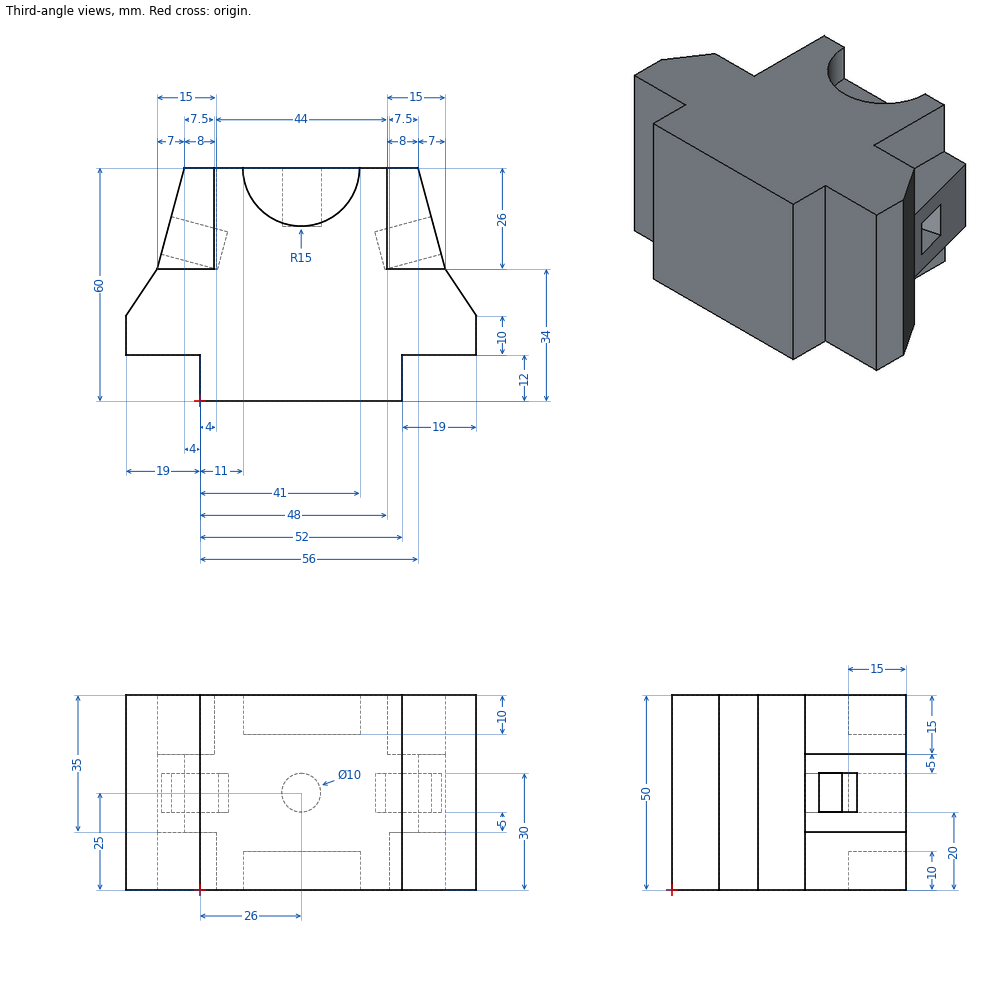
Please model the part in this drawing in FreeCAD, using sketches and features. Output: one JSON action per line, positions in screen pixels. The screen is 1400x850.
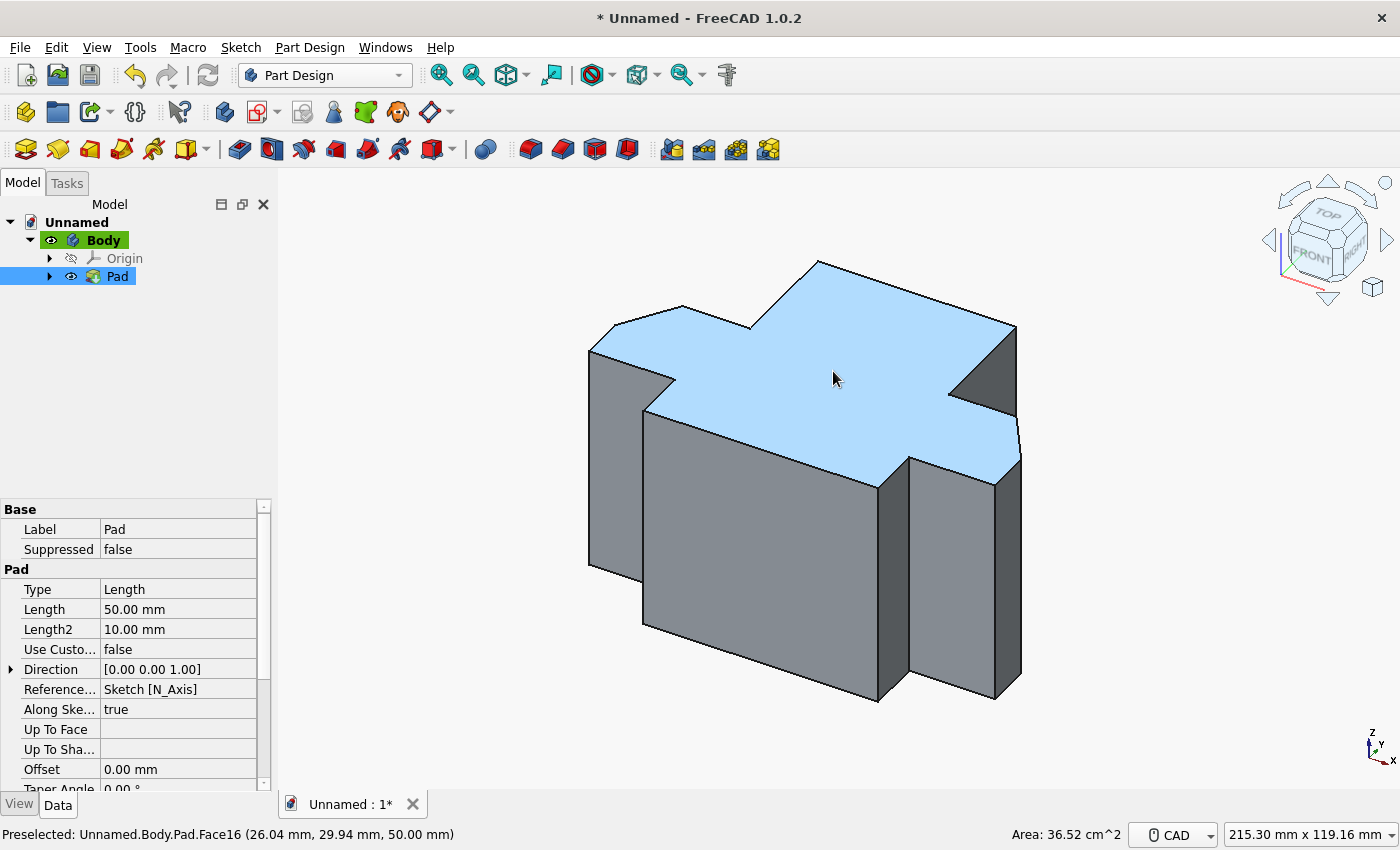
{"action": "left_click", "coordinate": [258, 112]}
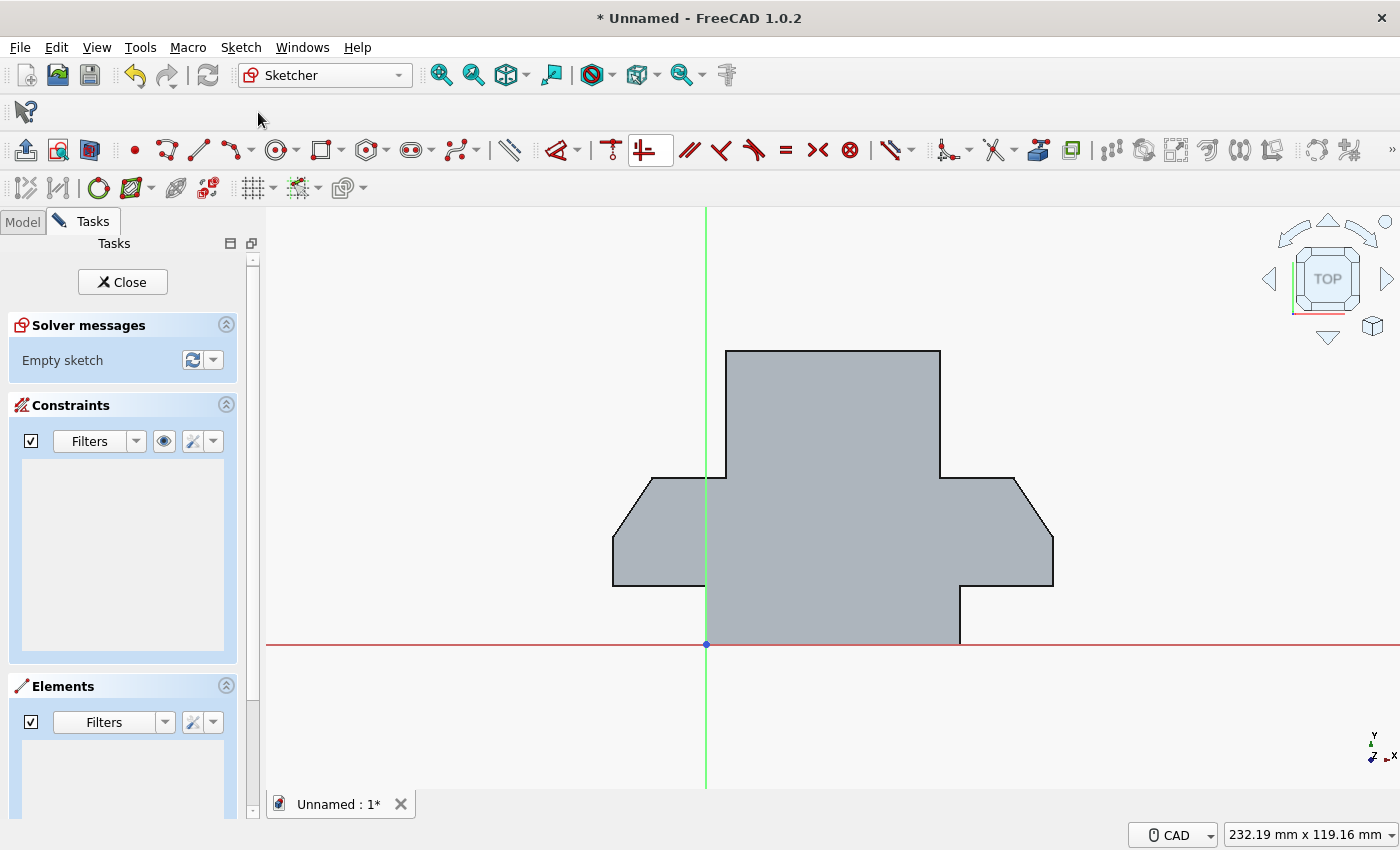
{"action": "left_click", "coordinate": [200, 150]}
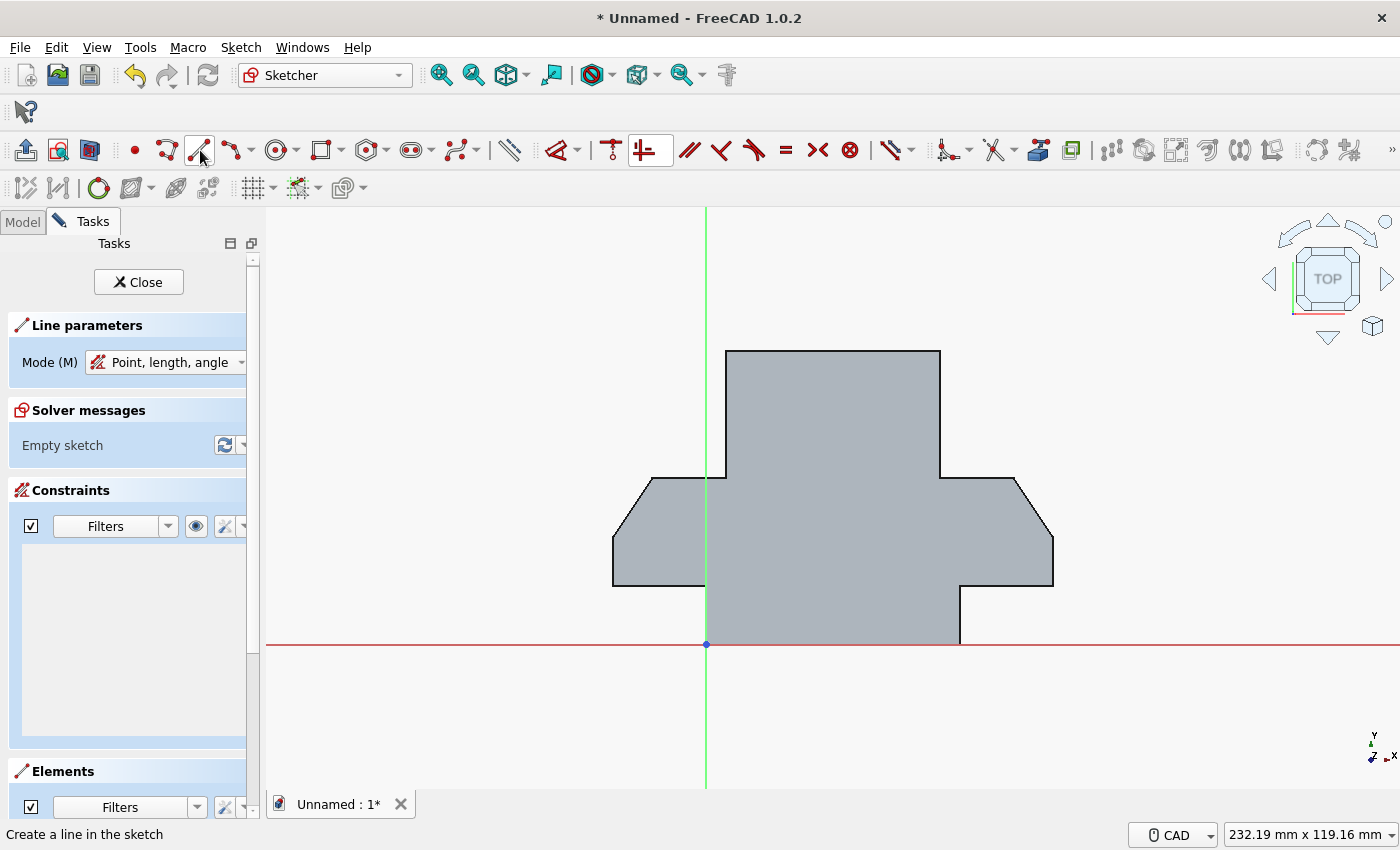
{"action": "left_click", "coordinate": [906, 351]}
{"action": "left_click", "coordinate": [760, 351]}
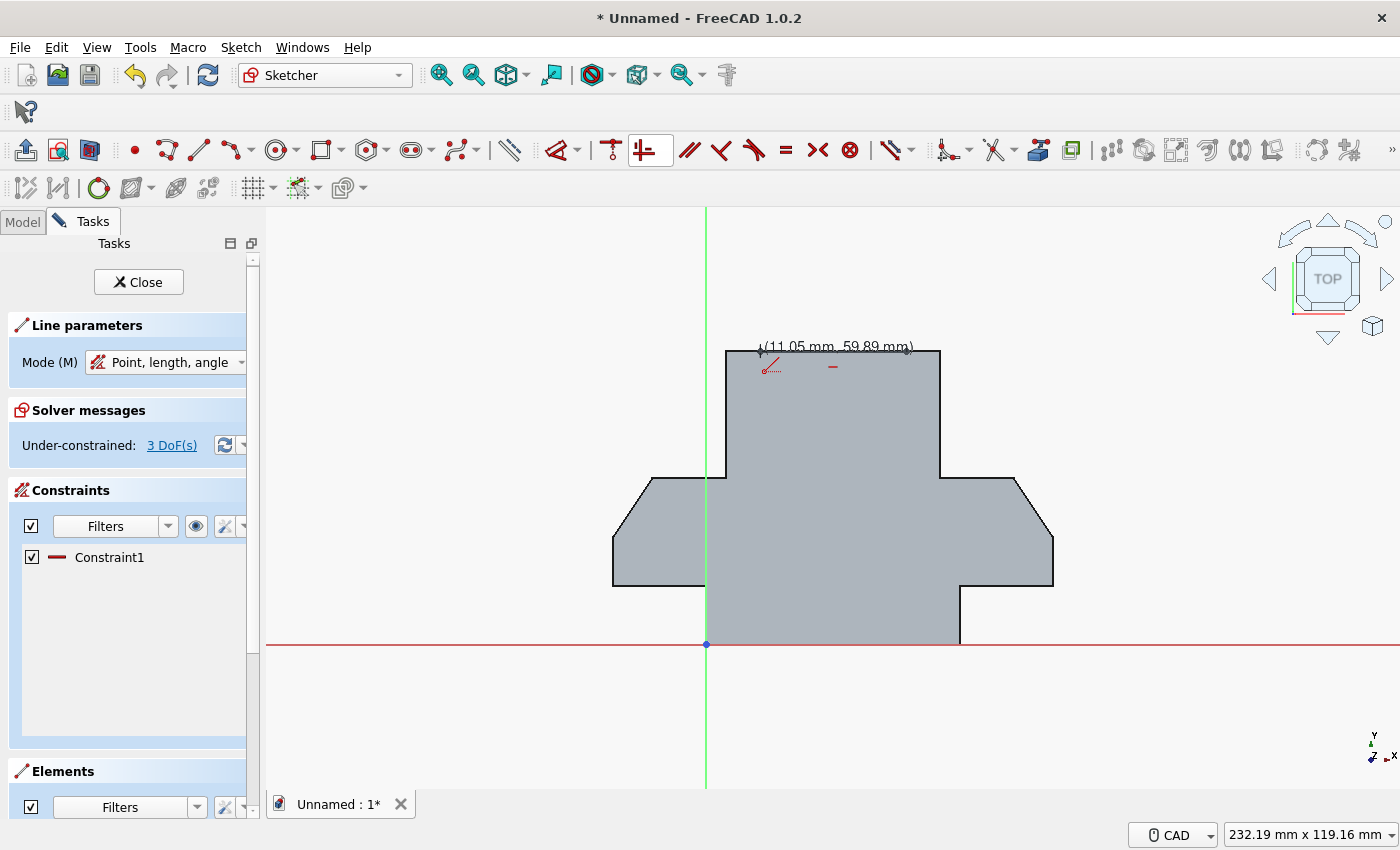
{"action": "left_click", "coordinate": [232, 150]}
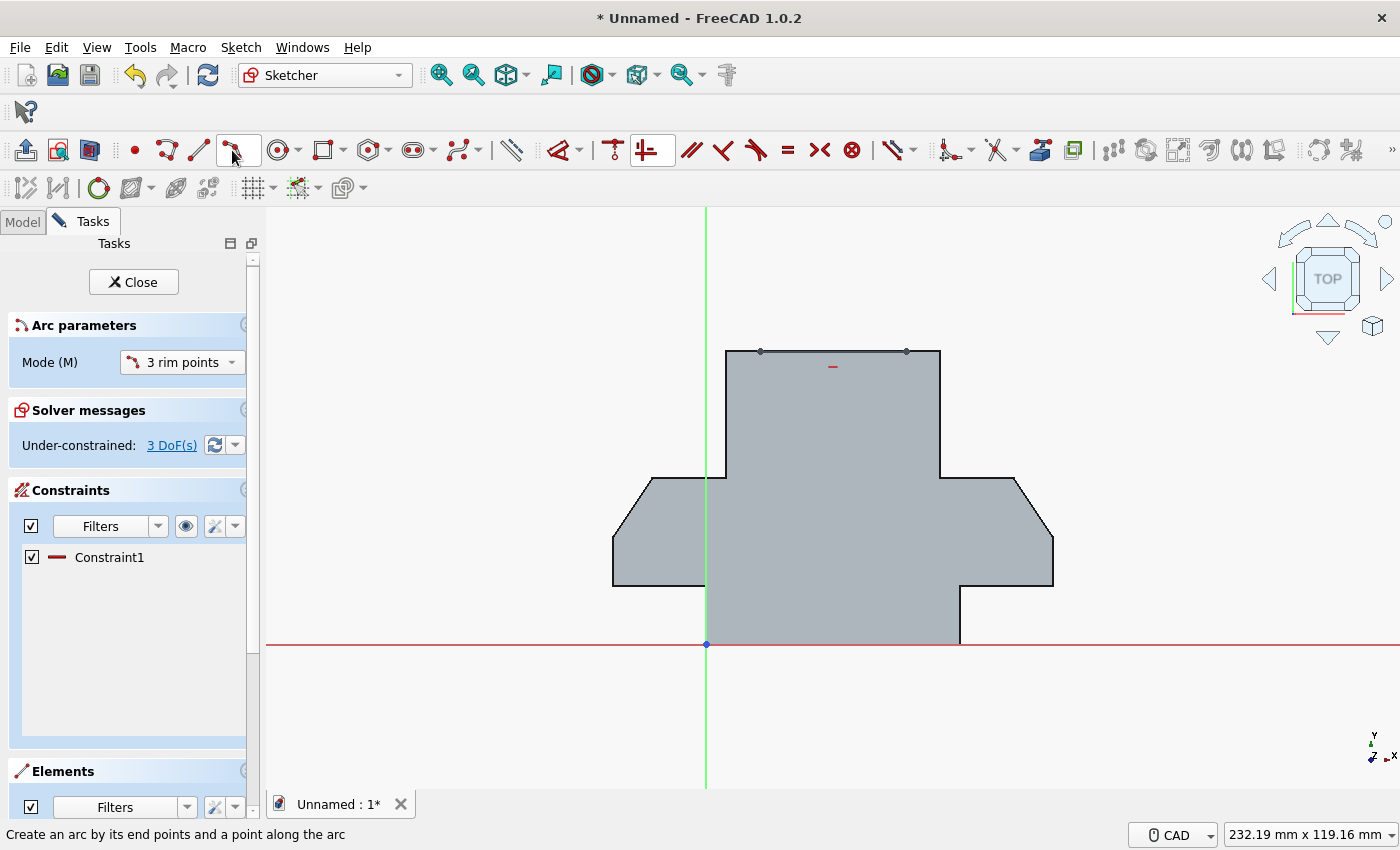
{"action": "left_click", "coordinate": [760, 352]}
{"action": "left_click", "coordinate": [906, 352]}
{"action": "left_click", "coordinate": [833, 425]}
{"action": "key", "text": "Escape"}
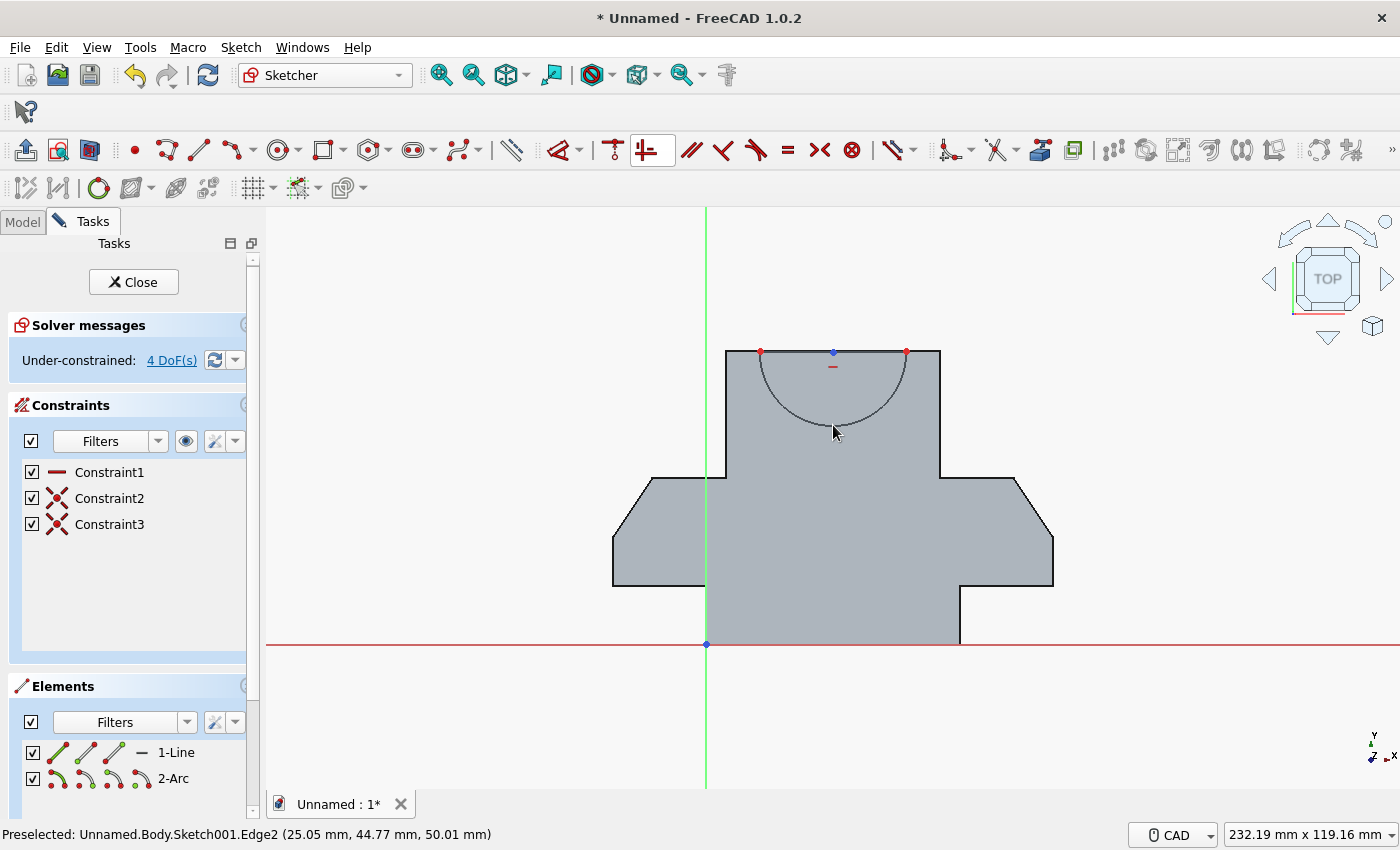
{"action": "left_click", "coordinate": [558, 150]}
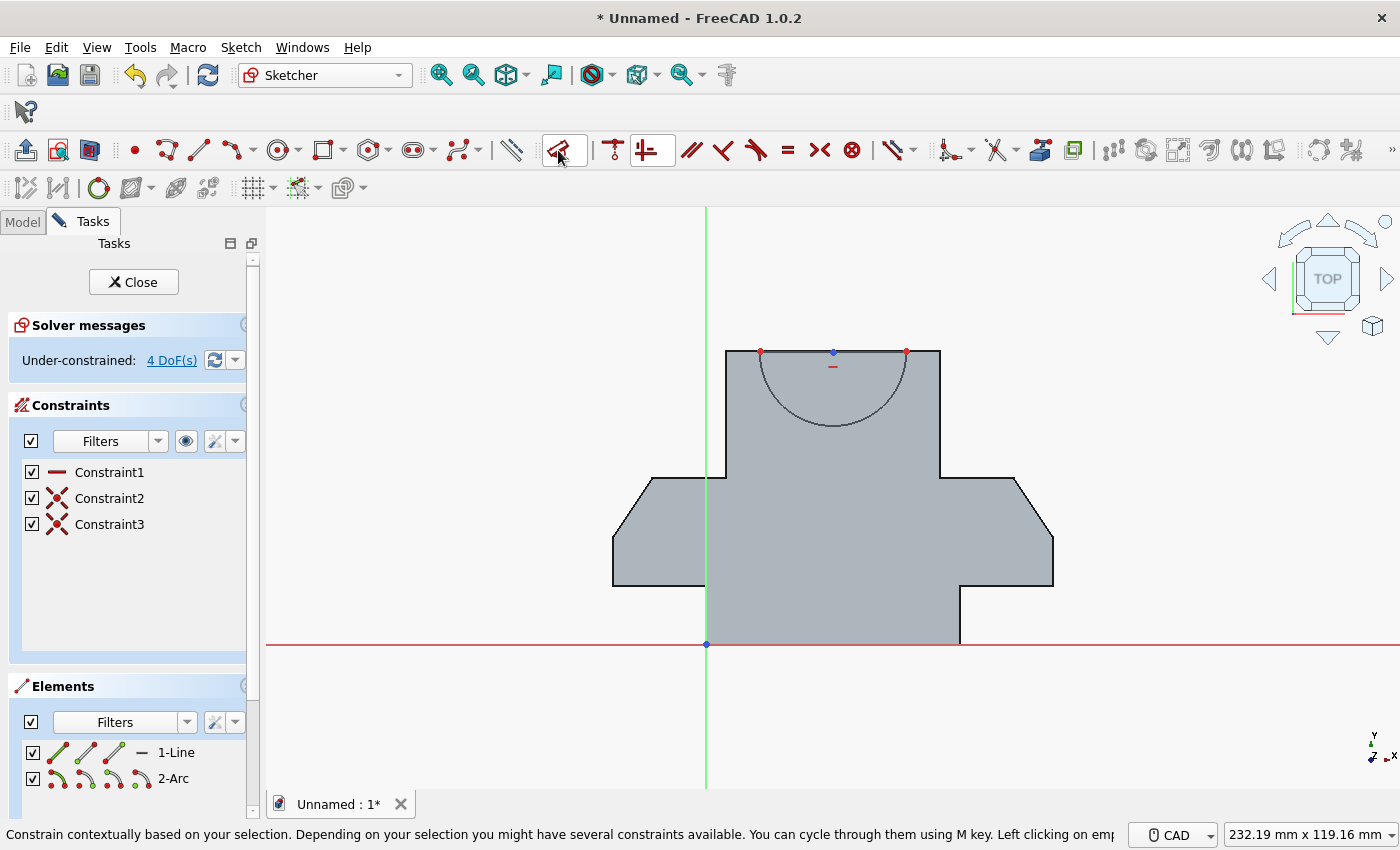
{"action": "left_click", "coordinate": [790, 412]}
{"action": "left_click", "coordinate": [771, 438]}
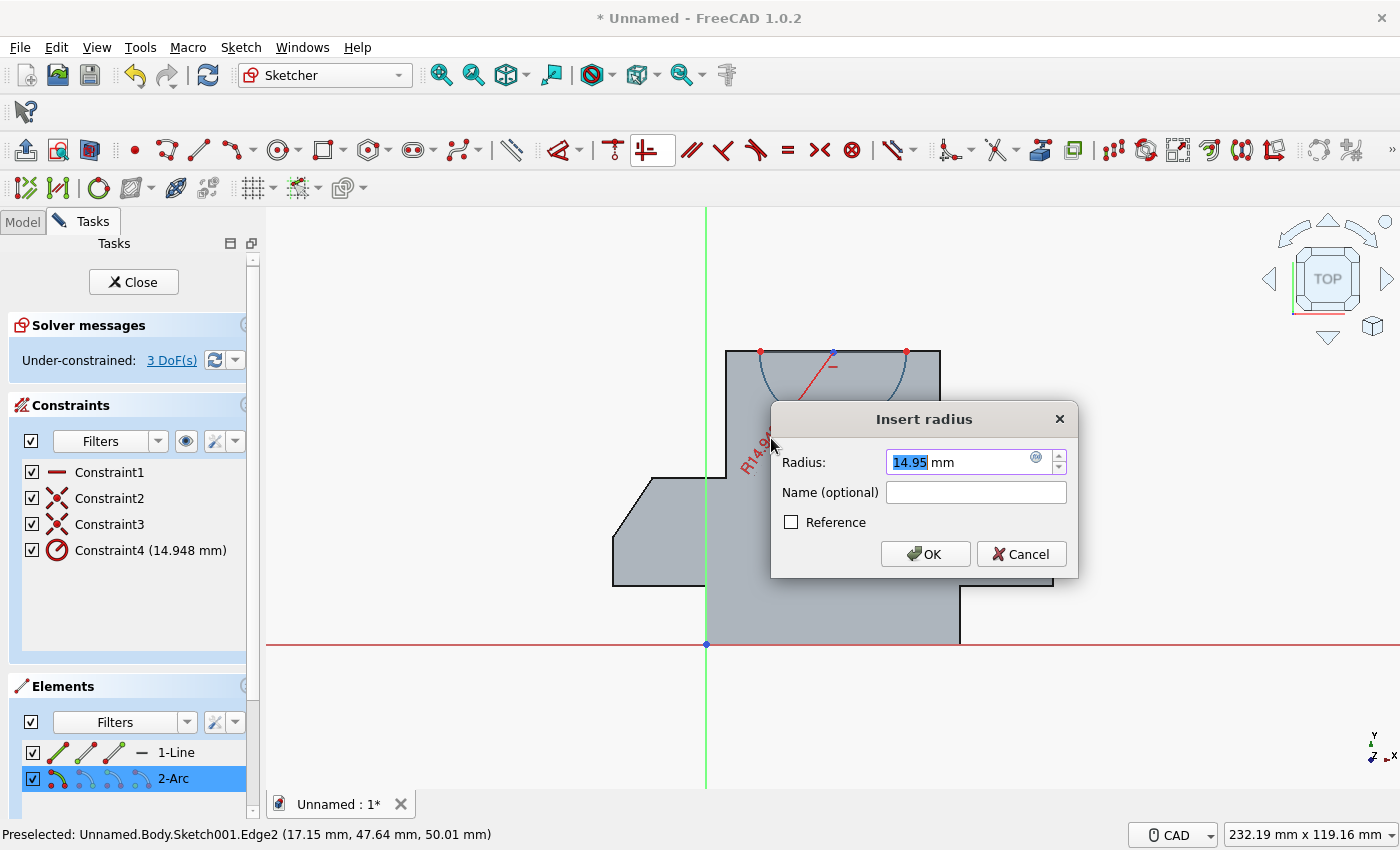
{"action": "type", "text": "15"}
{"action": "key", "text": "Return"}